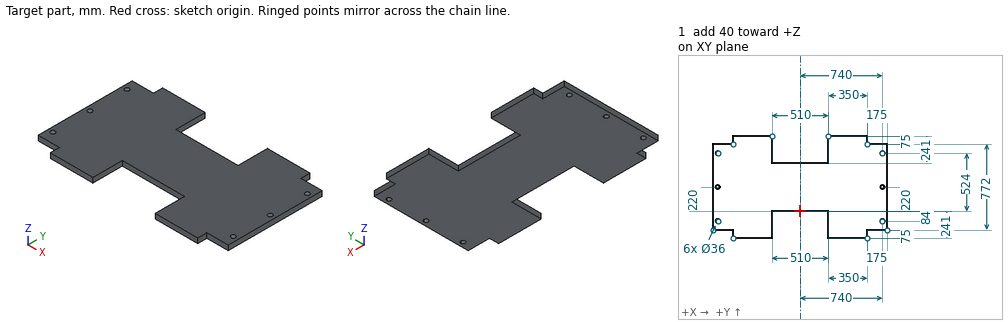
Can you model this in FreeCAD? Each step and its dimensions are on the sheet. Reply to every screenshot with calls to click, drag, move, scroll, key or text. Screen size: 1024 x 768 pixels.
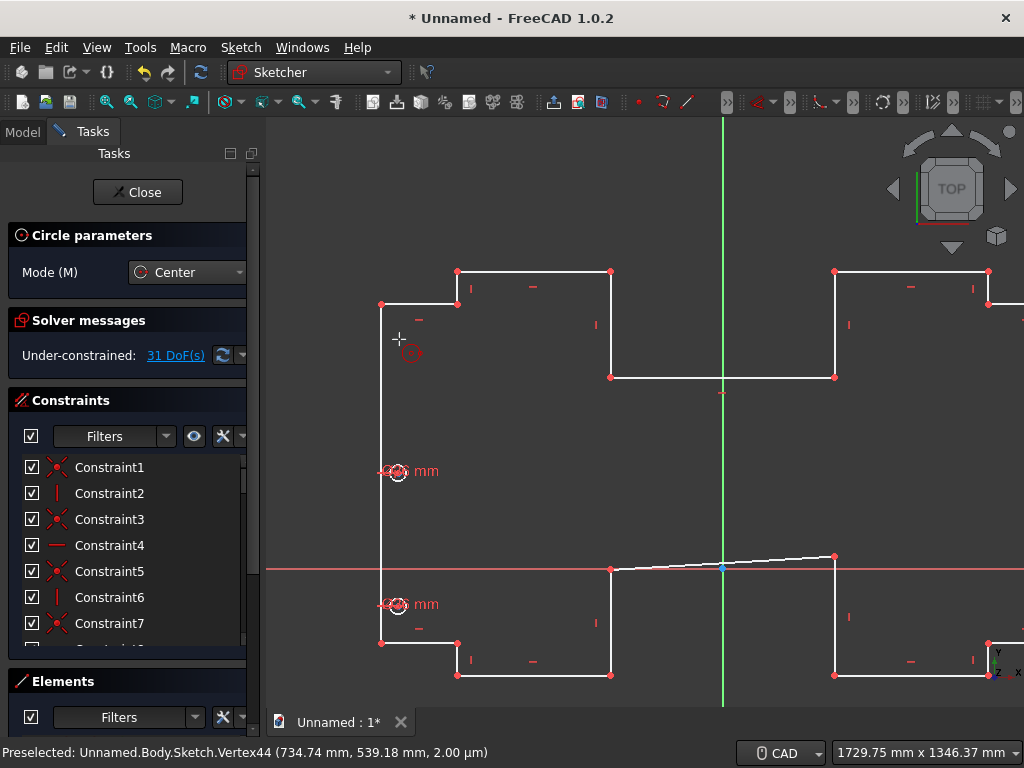
click(398, 339)
move(404, 334)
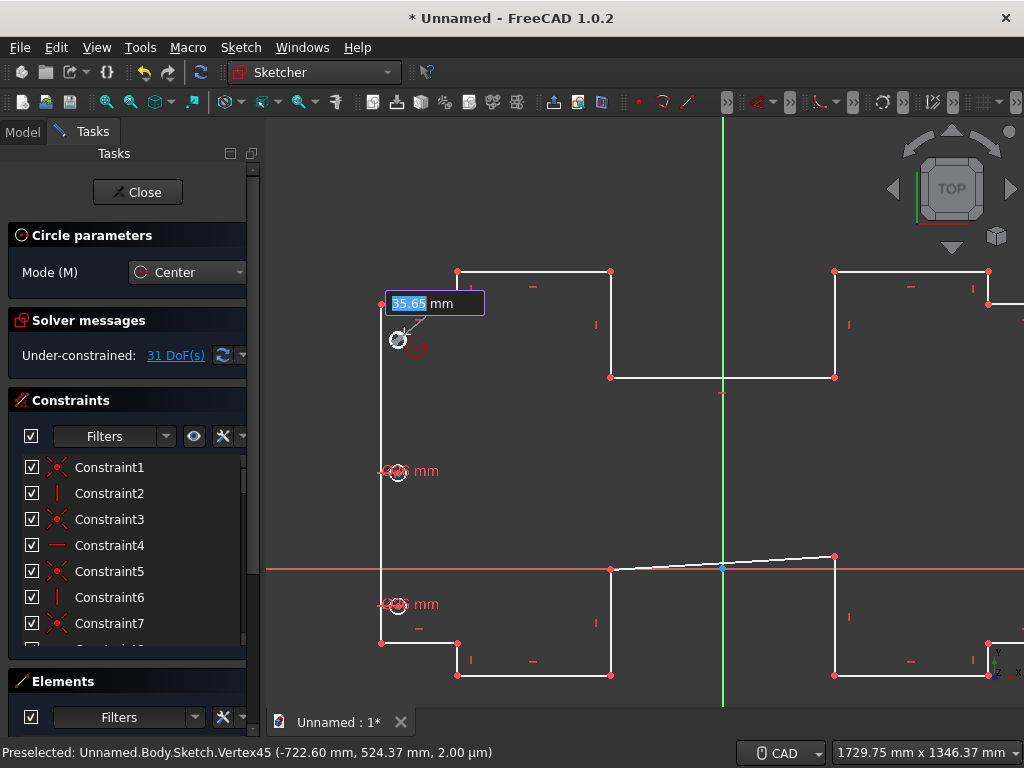
text(36)
key(Return)
key(Escape)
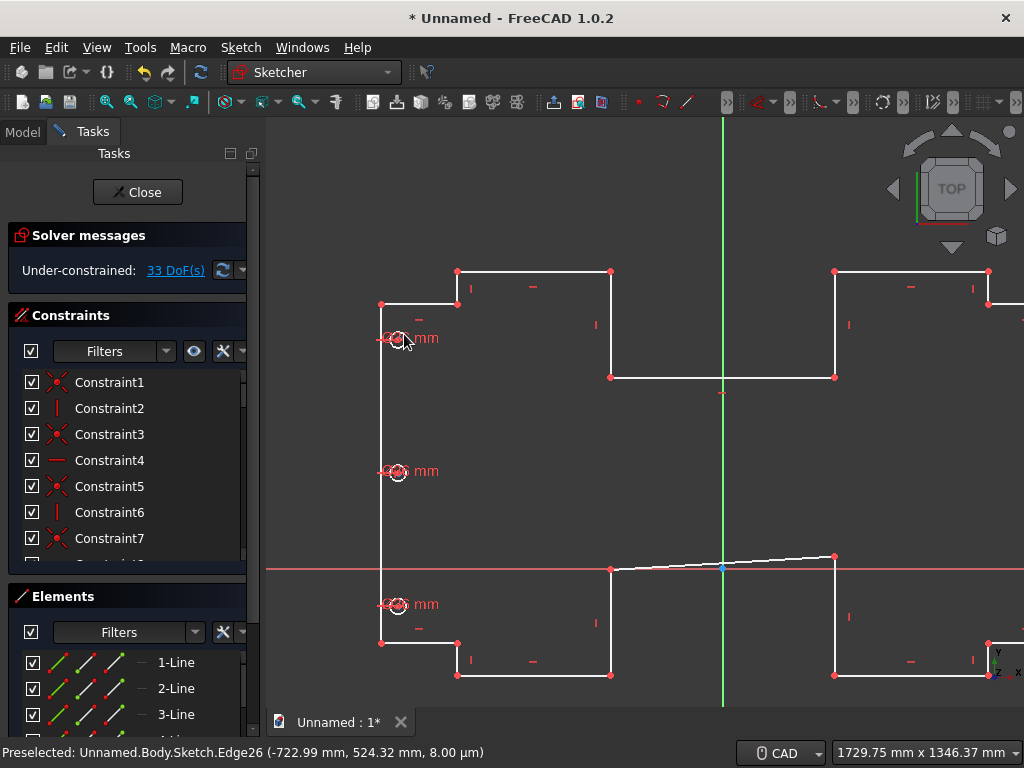
click(678, 566)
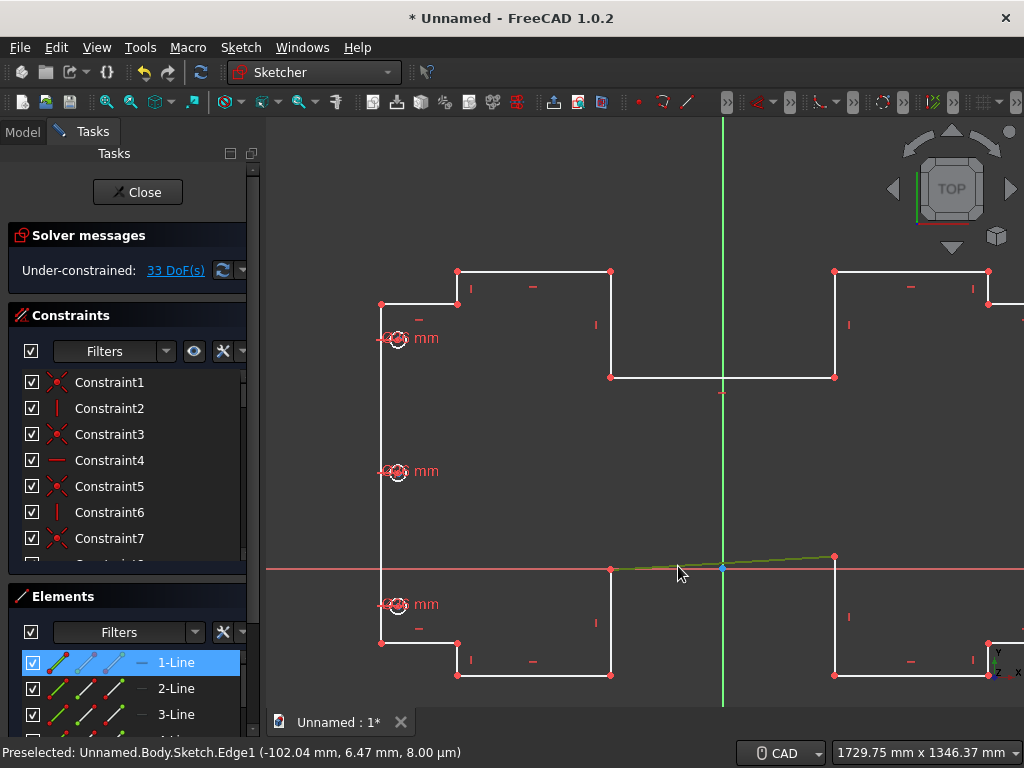
key(h)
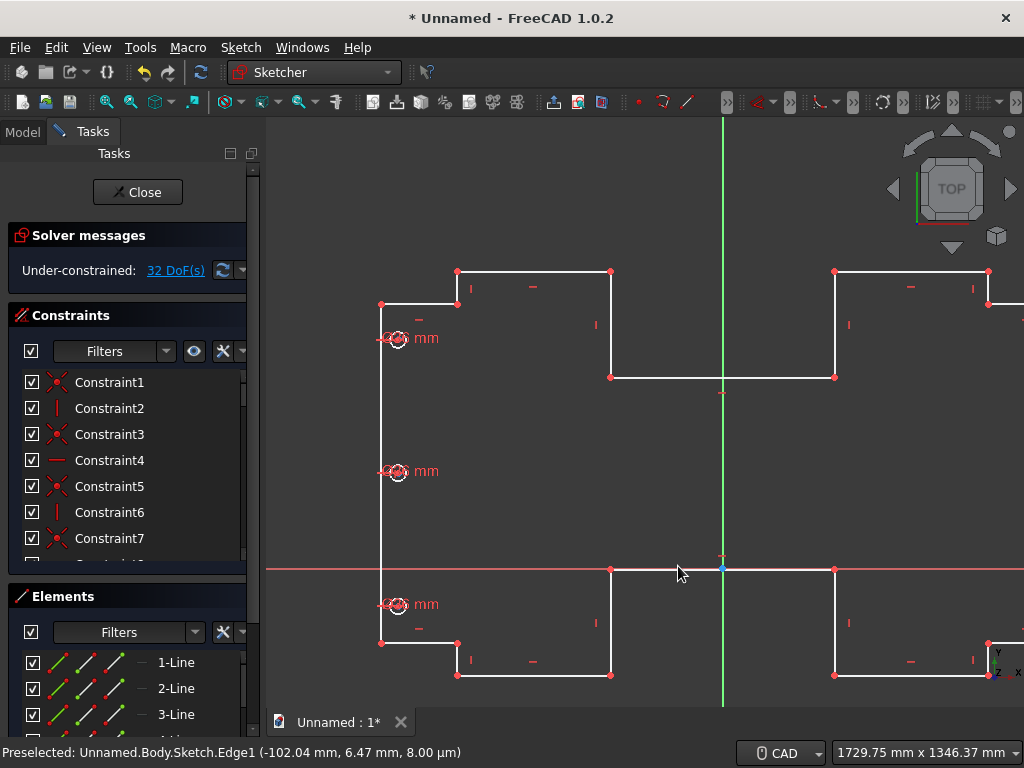
scroll(399, 339, down, 3)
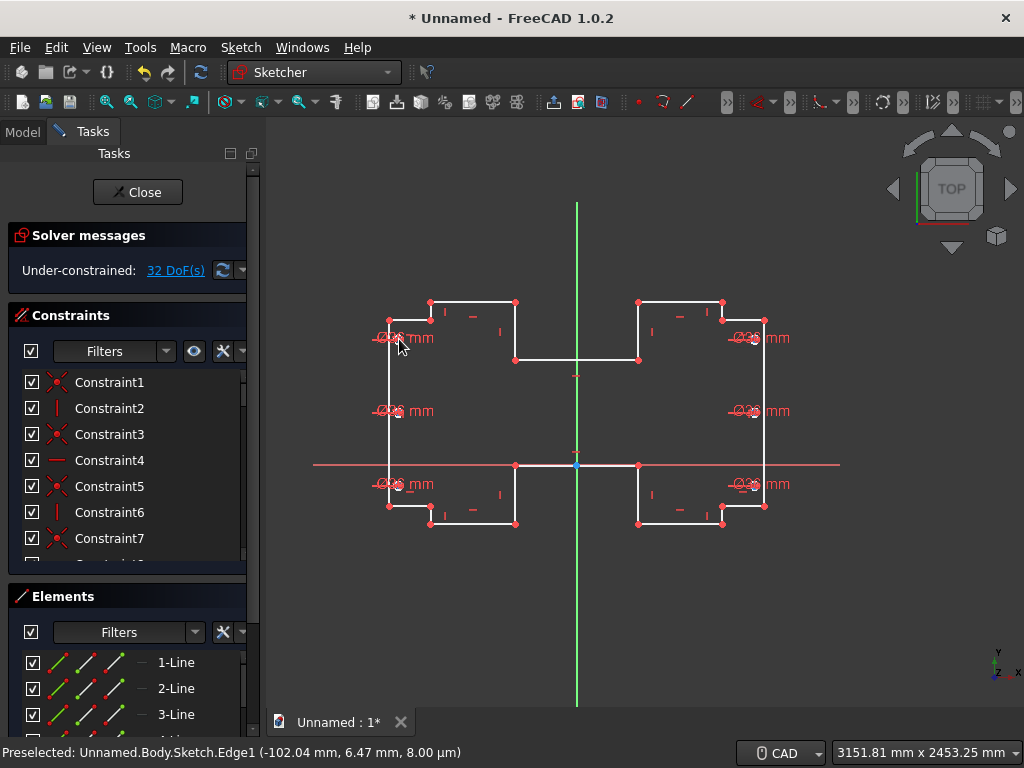
click(755, 486)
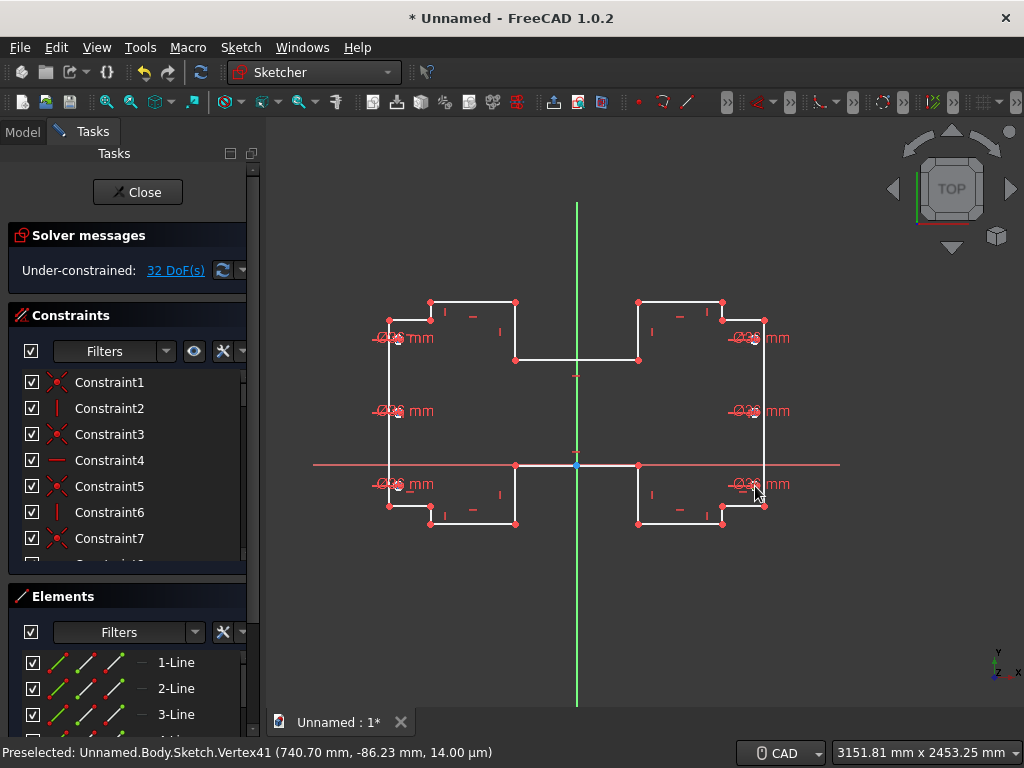
click(755, 413)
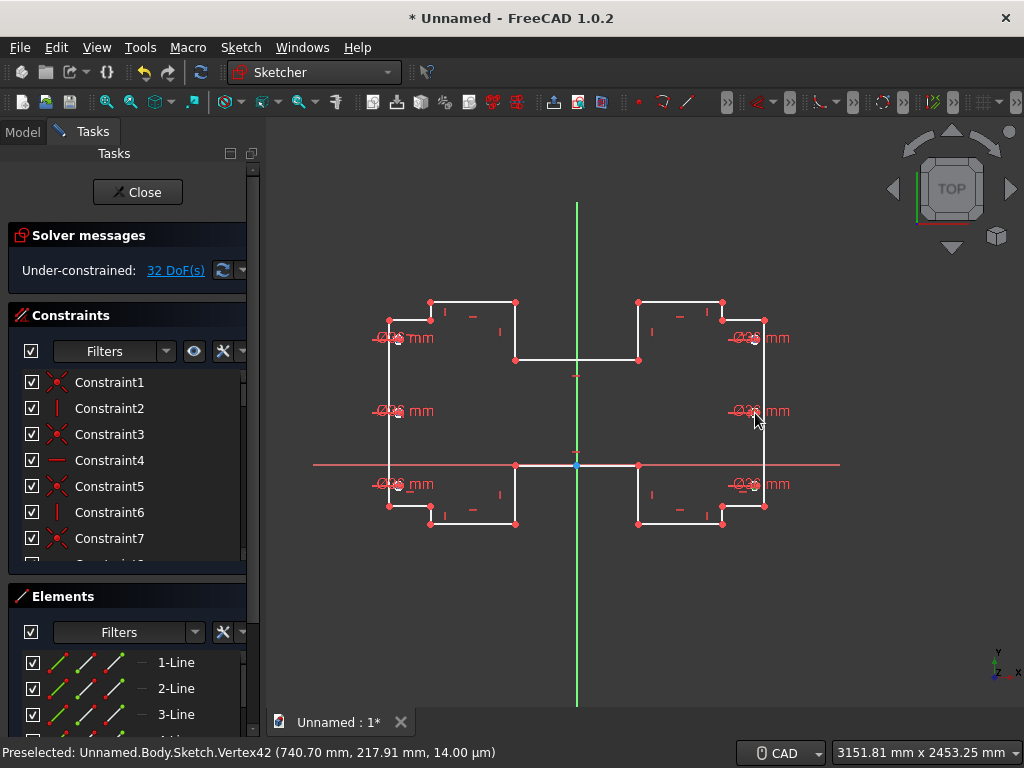
key(v)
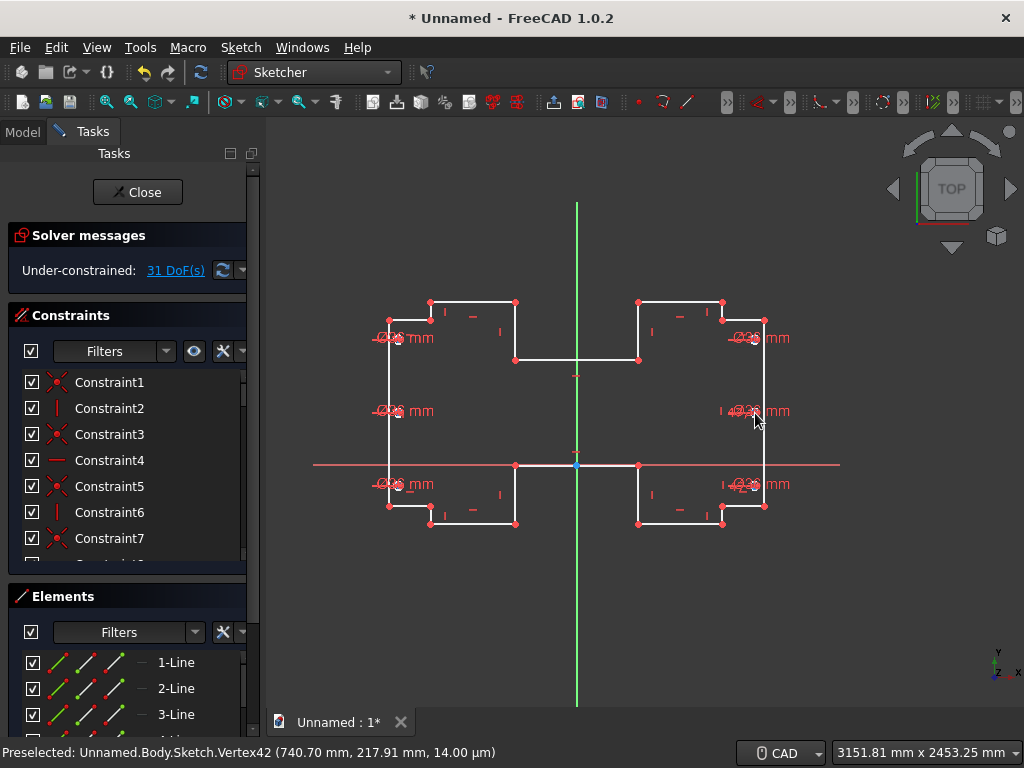
click(399, 486)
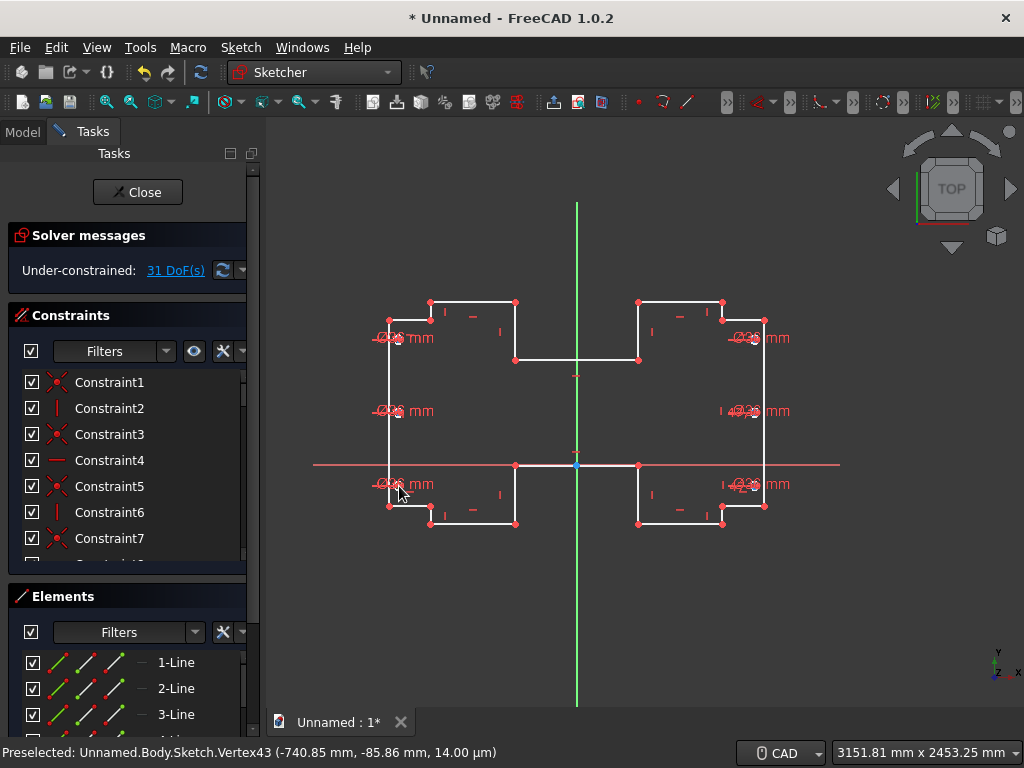
click(399, 413)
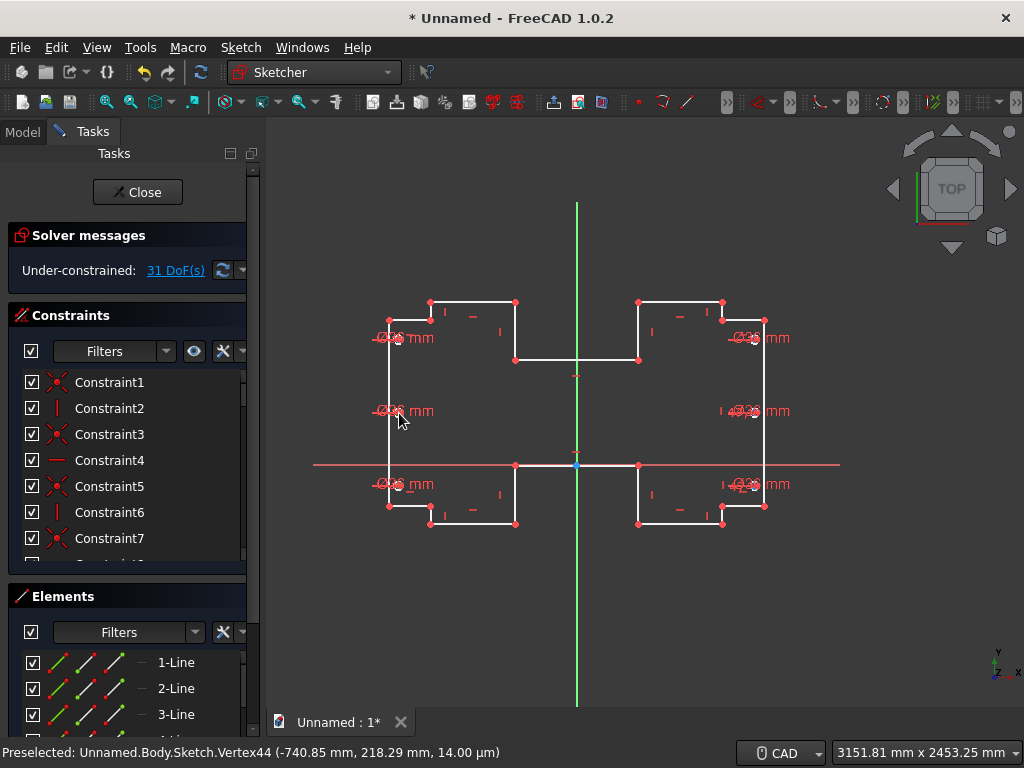
key(v)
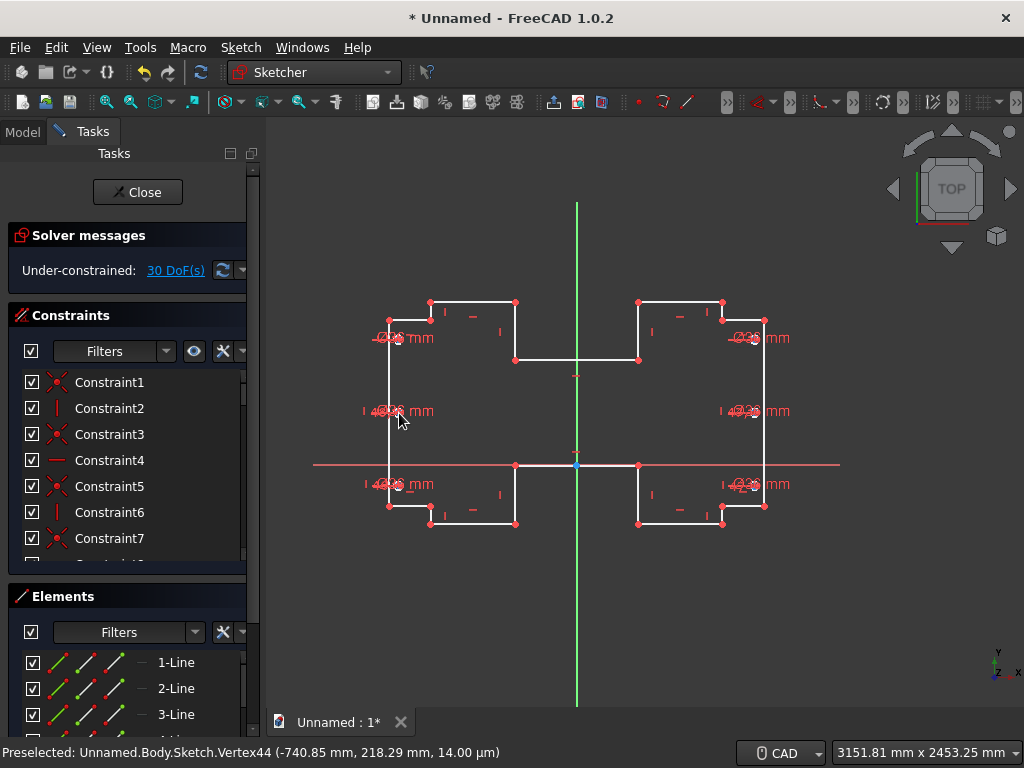
click(755, 486)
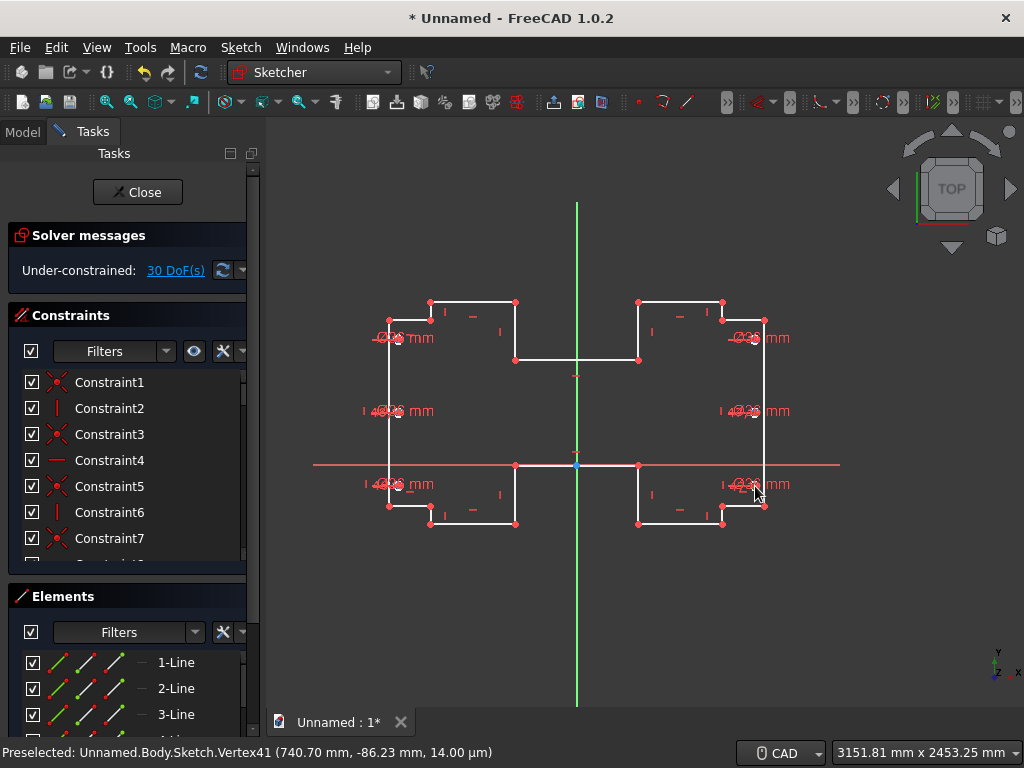
click(399, 486)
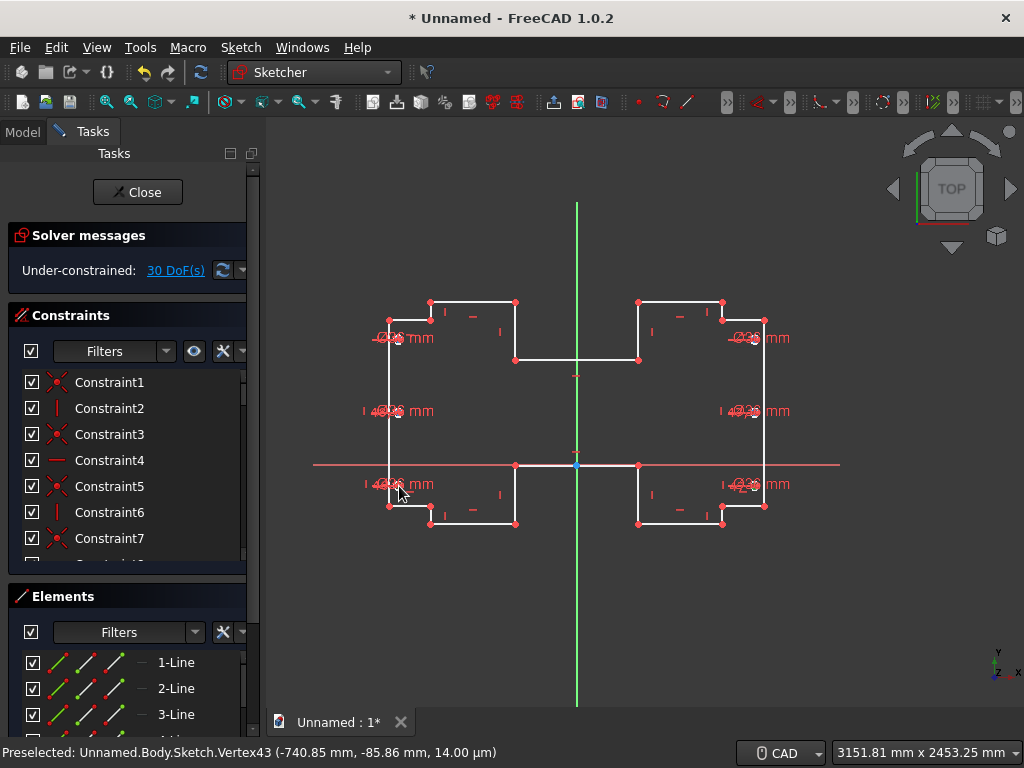
click(577, 641)